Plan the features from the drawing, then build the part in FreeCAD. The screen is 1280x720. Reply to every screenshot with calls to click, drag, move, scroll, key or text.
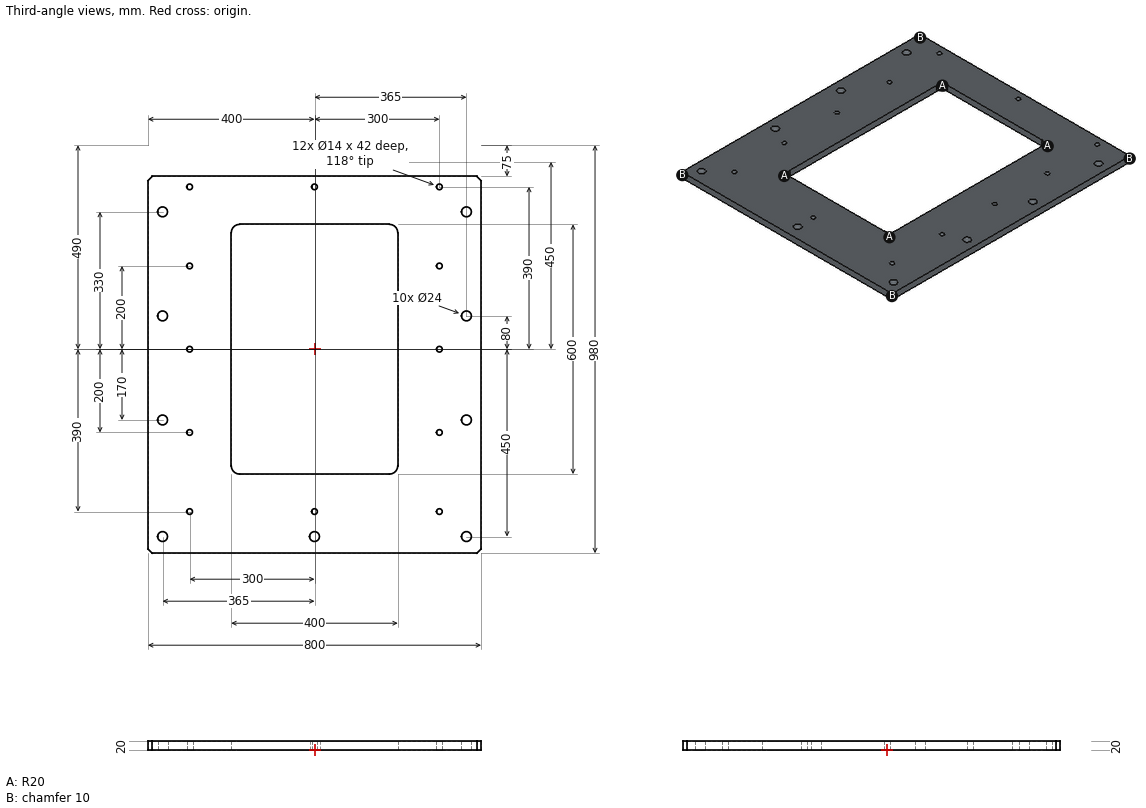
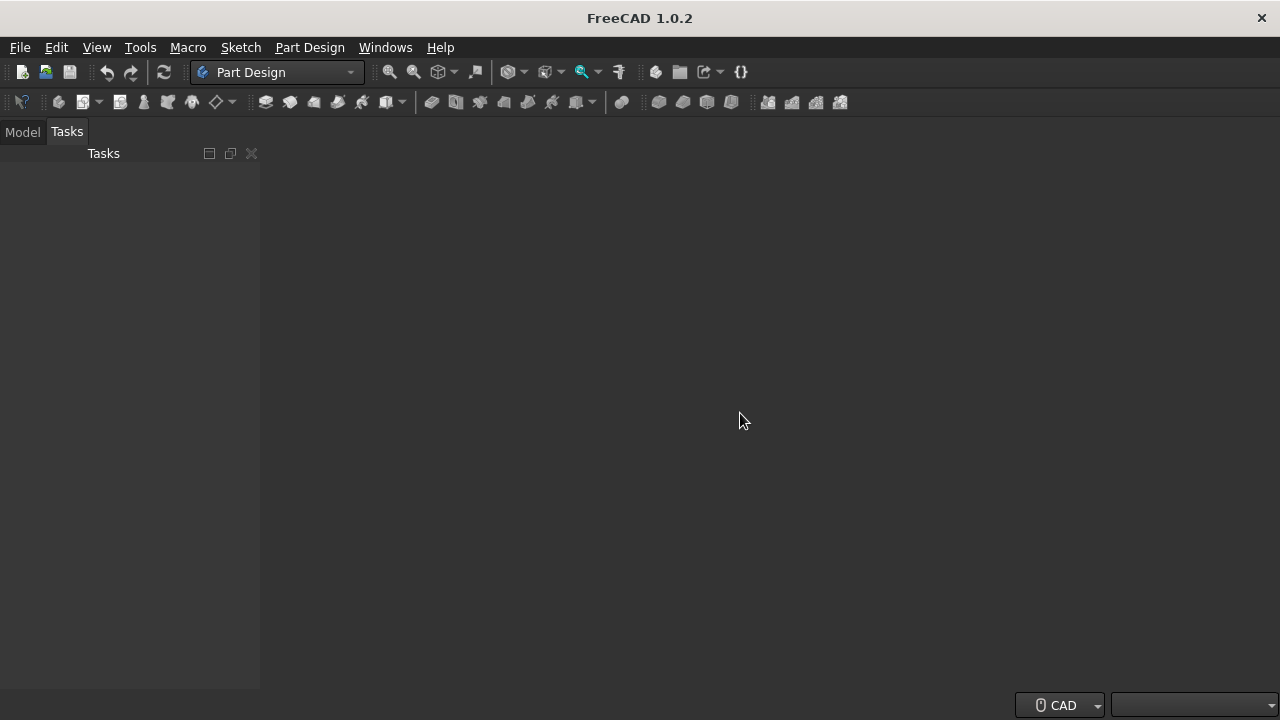
click(22, 72)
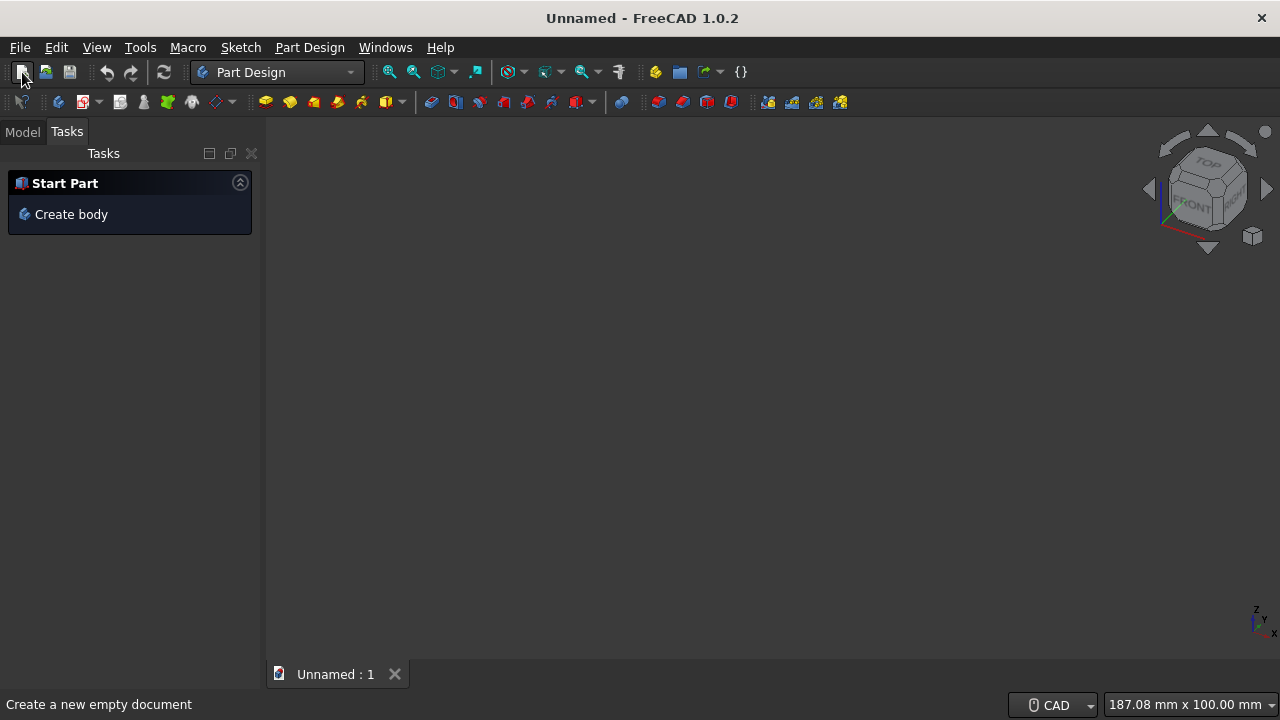
click(84, 102)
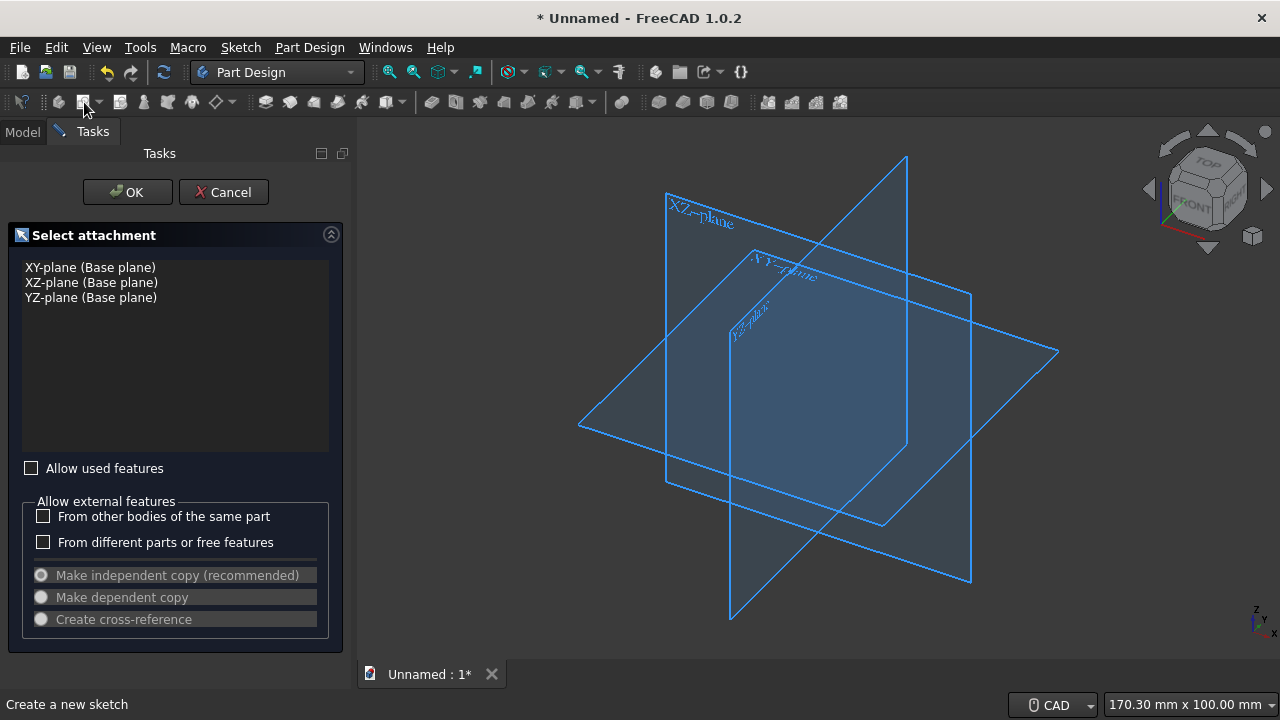
click(82, 268)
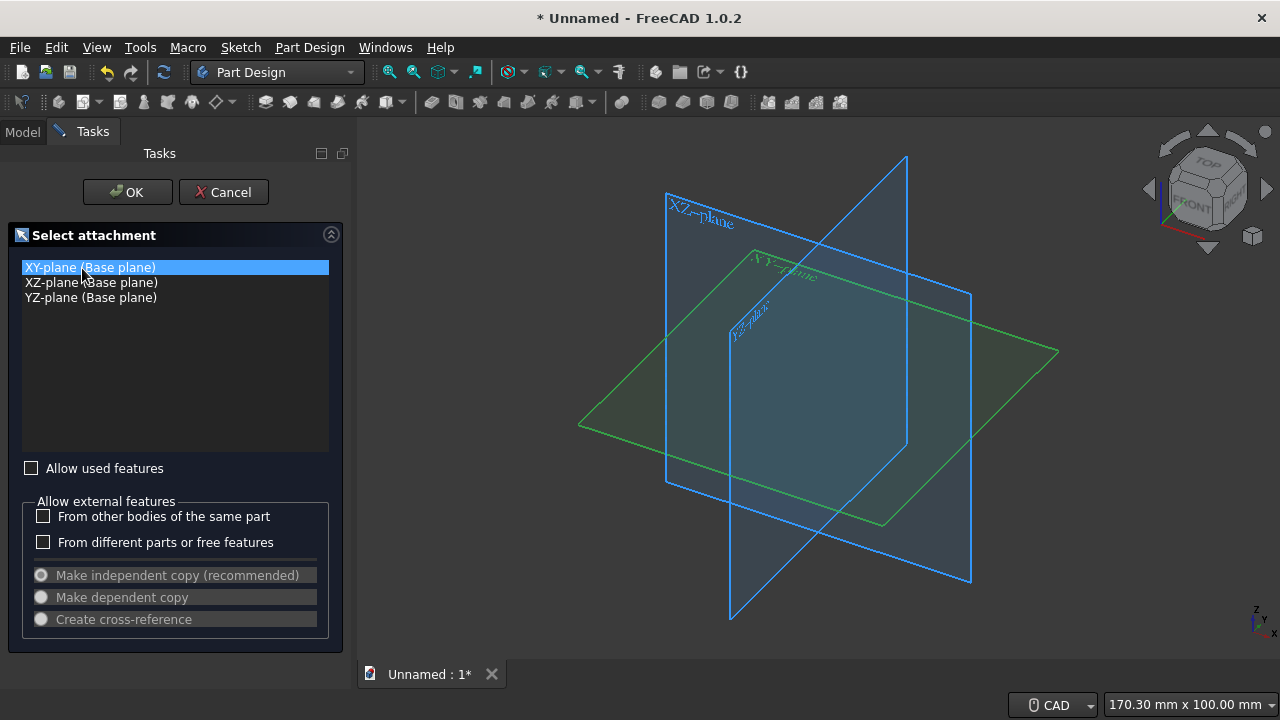
click(128, 192)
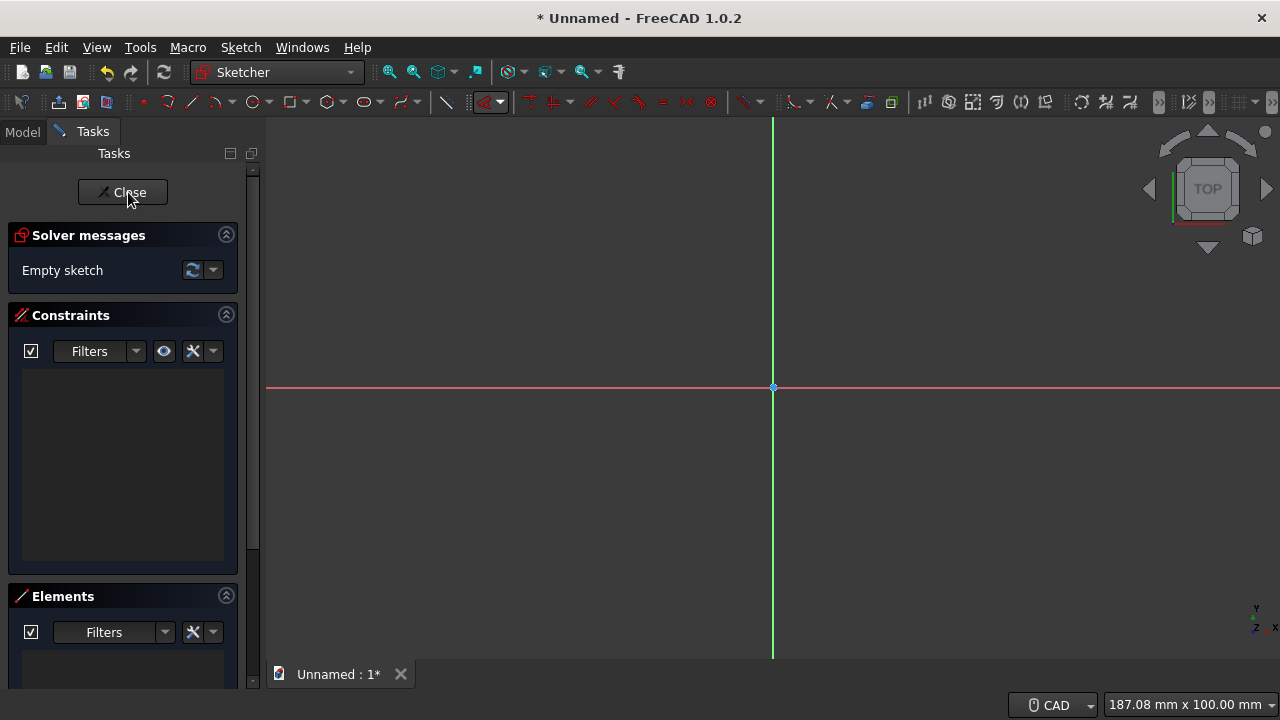
scroll(700, 388, down, 14)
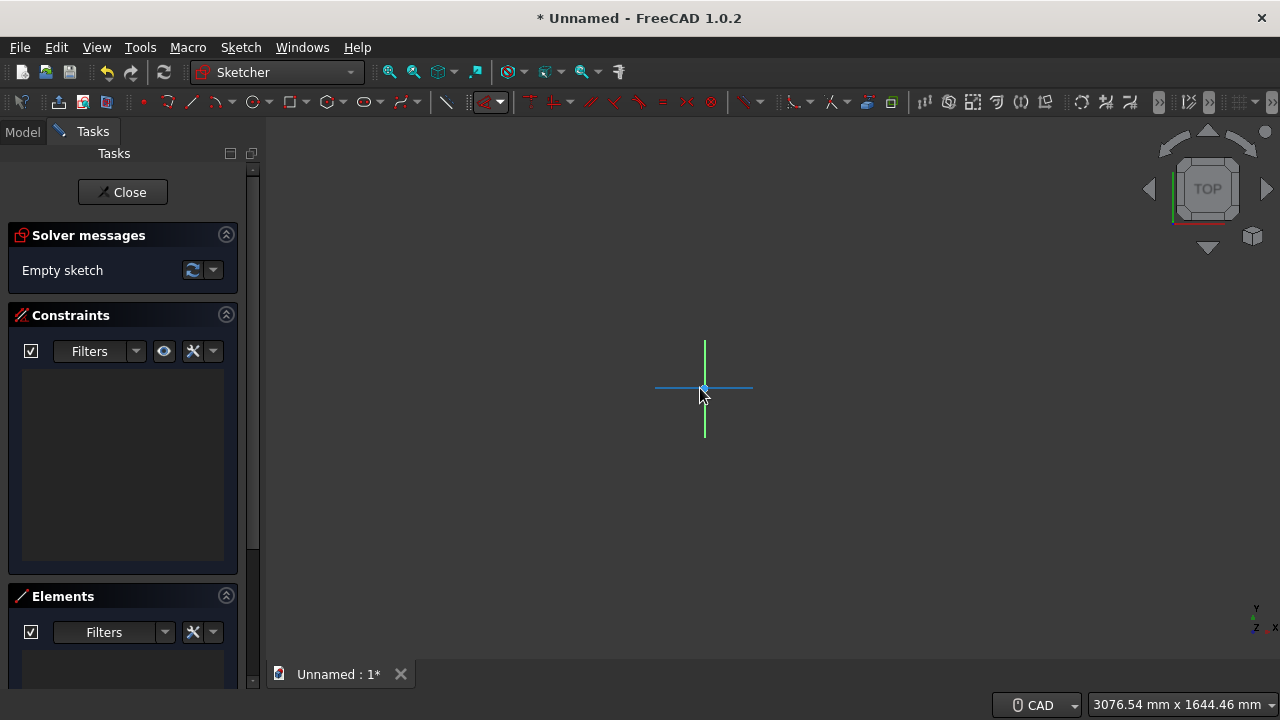
click(308, 102)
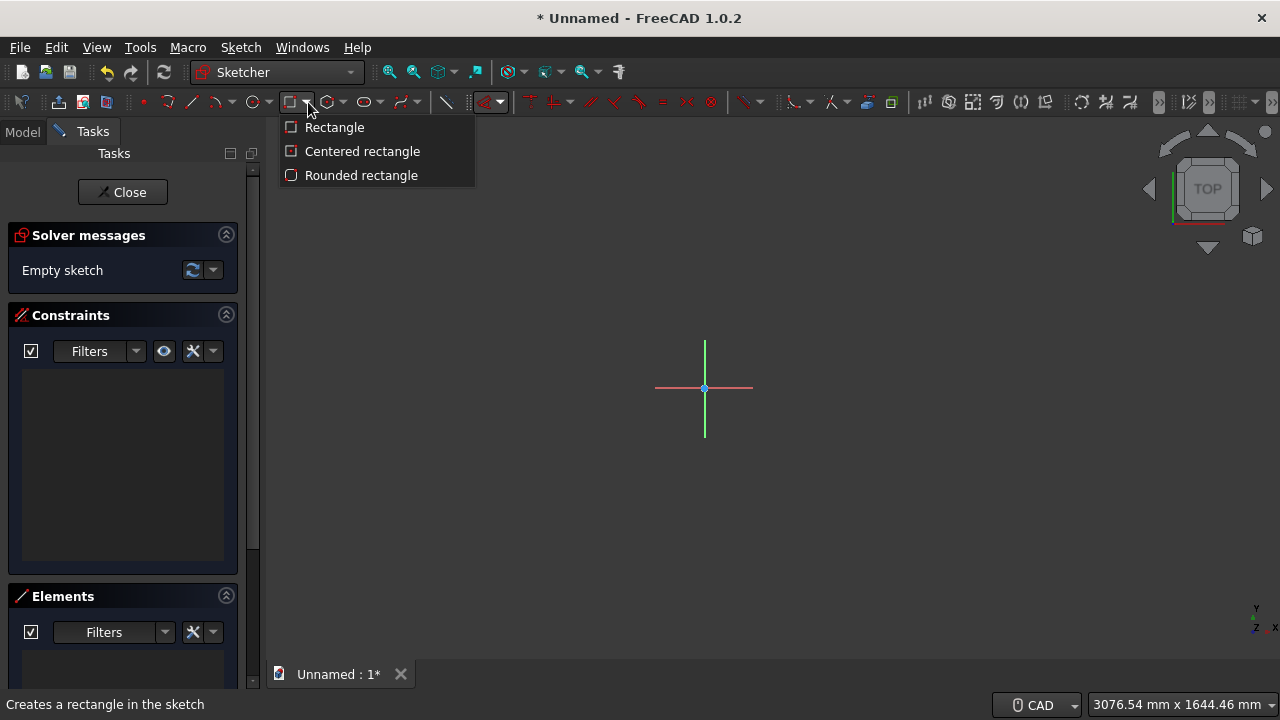
click(378, 151)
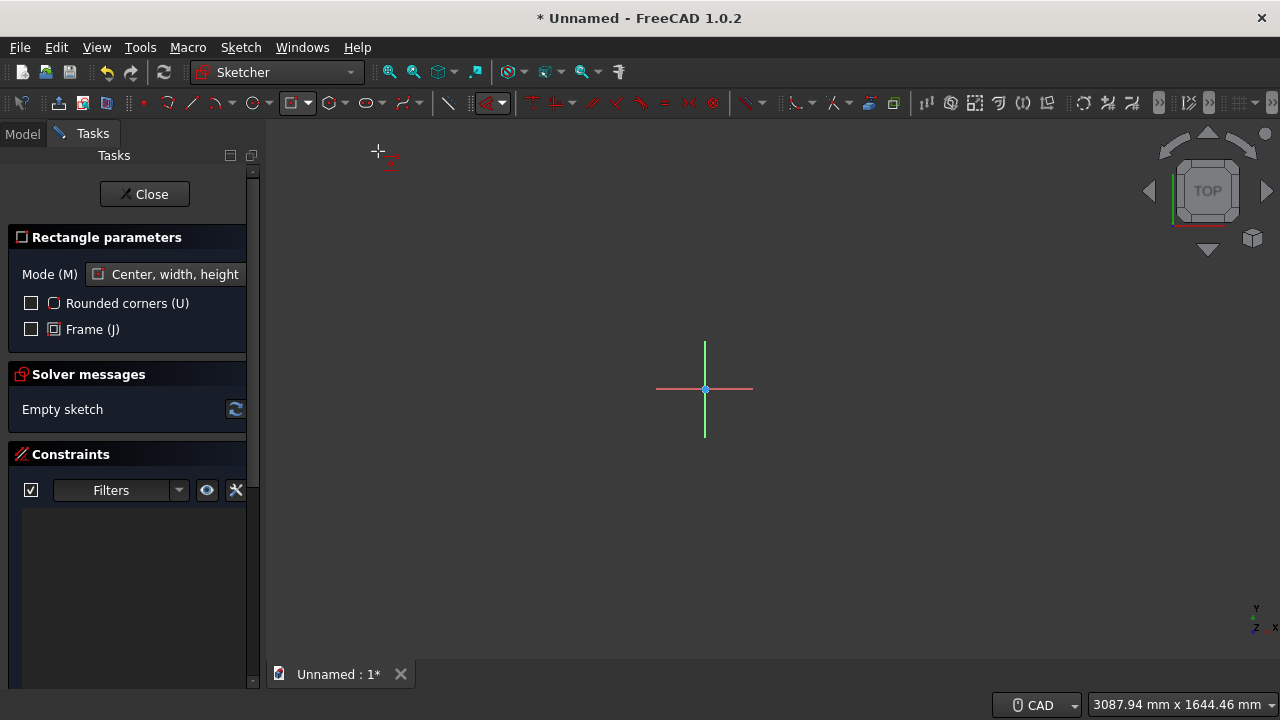
click(705, 389)
move(836, 229)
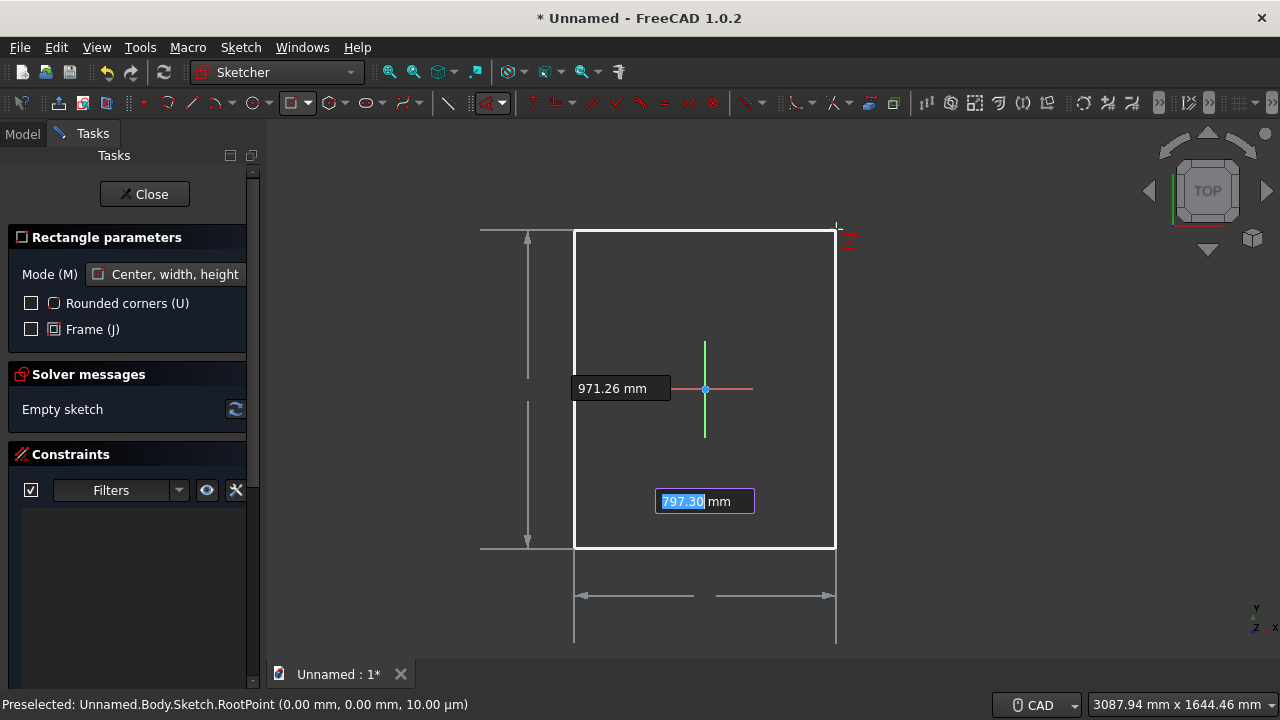
text(800)
key(Tab)
text(980)
key(Return)
key(Escape)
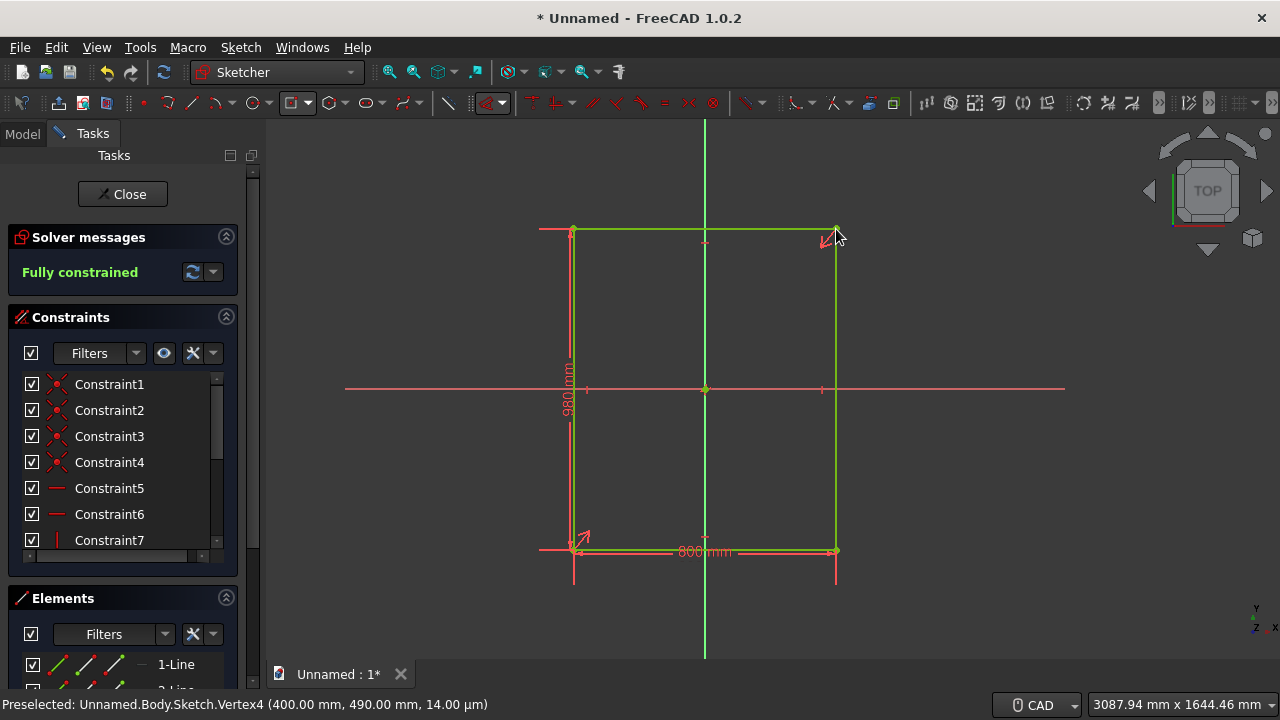
click(123, 194)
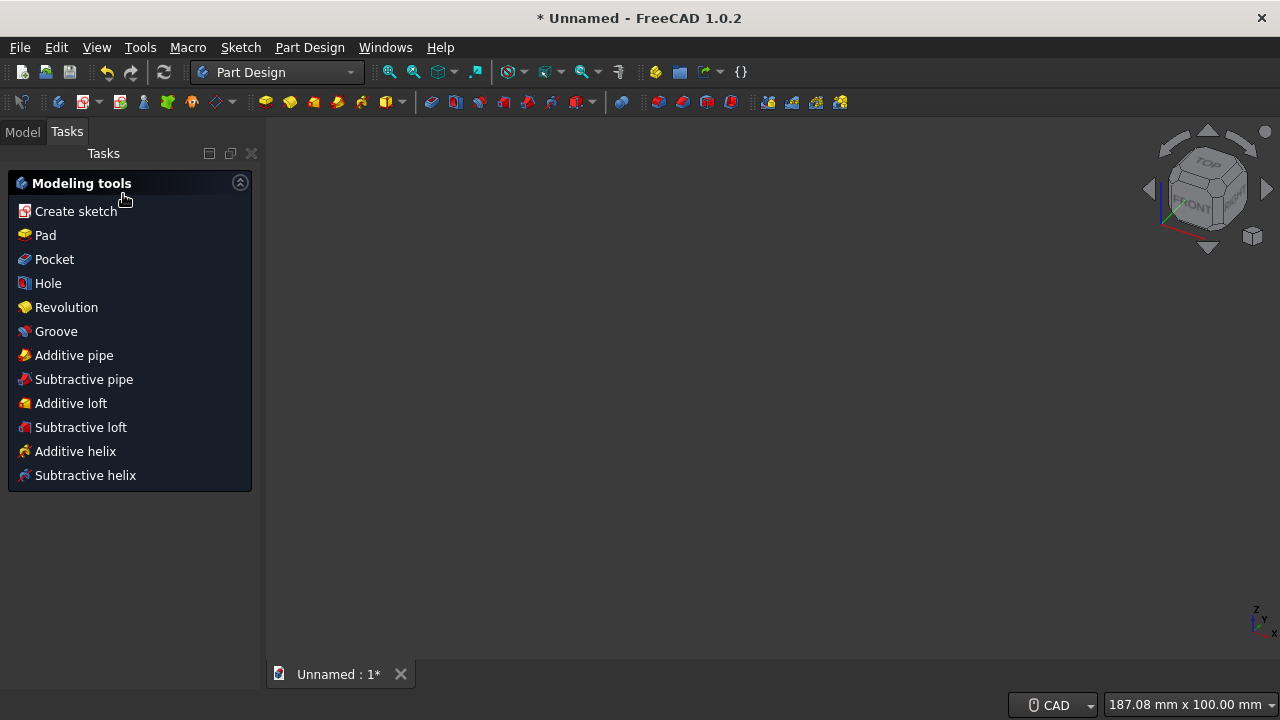
click(266, 102)